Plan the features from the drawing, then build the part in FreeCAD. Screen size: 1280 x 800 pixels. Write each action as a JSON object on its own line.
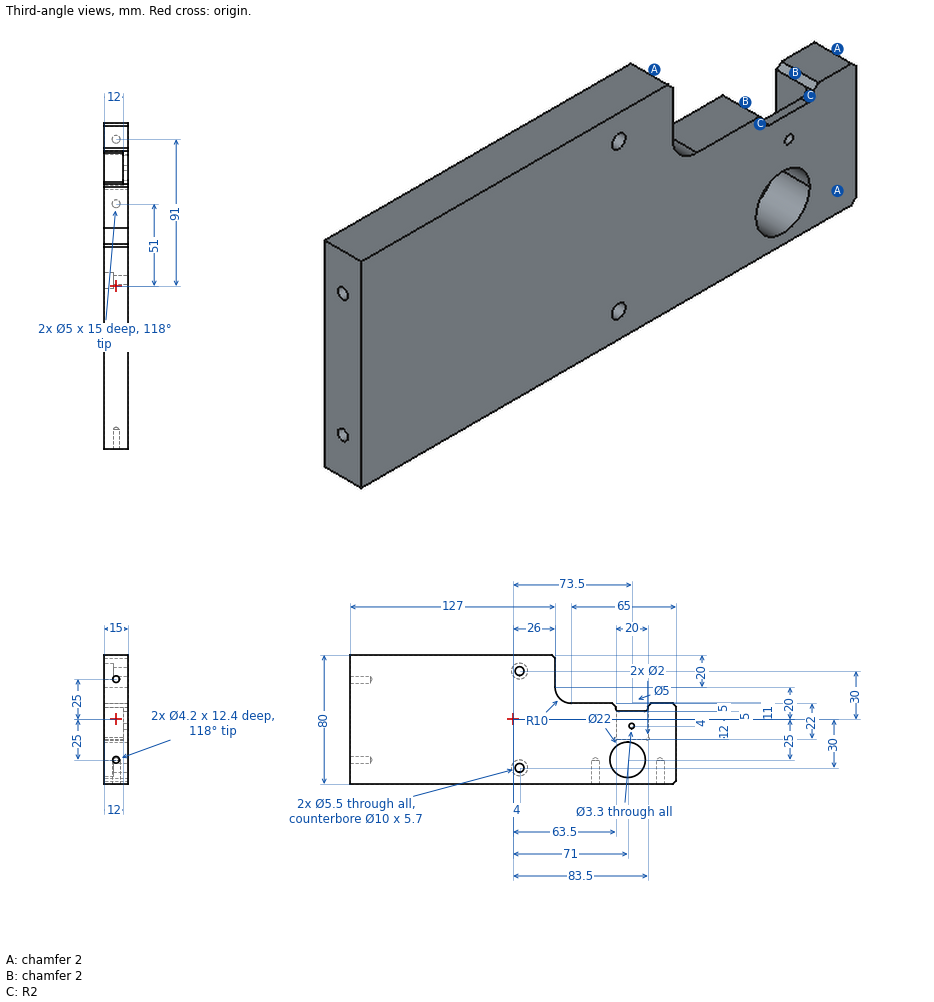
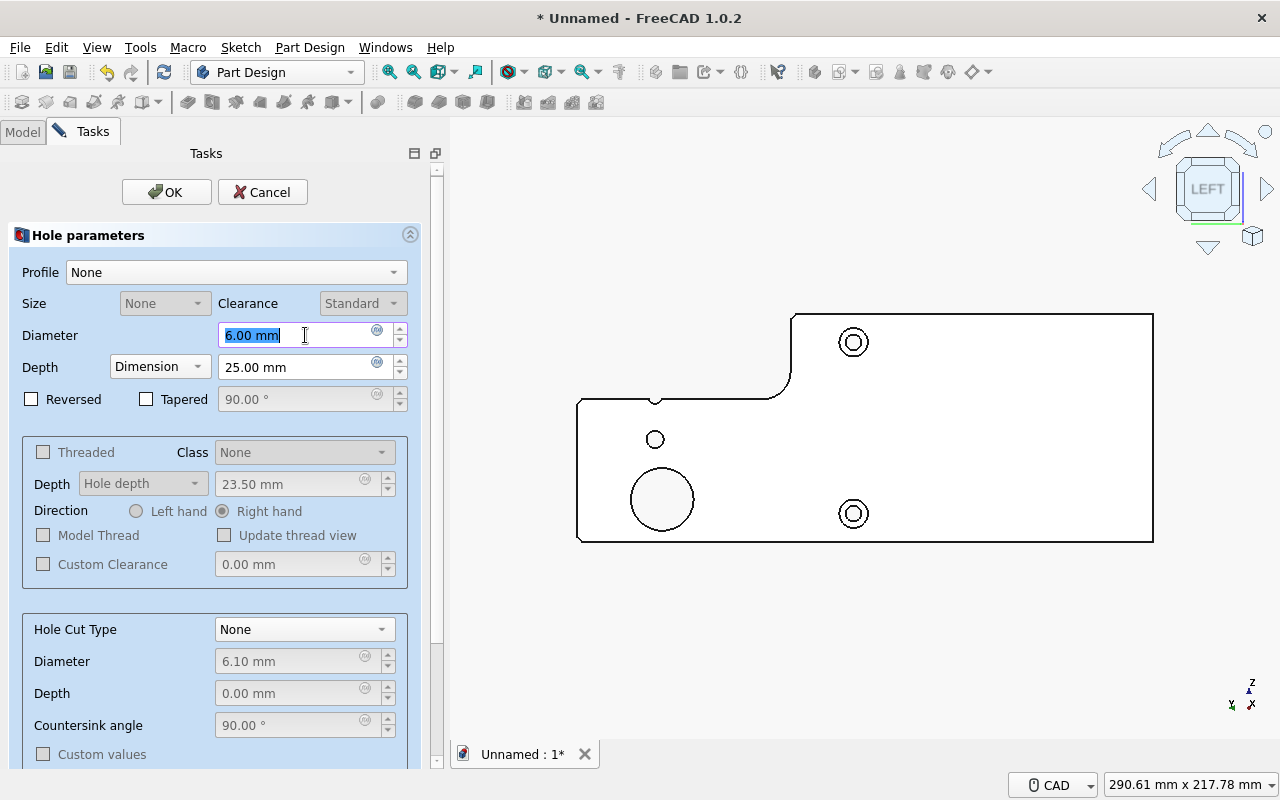
{"action": "type", "text": "3.3"}
{"action": "key", "text": "Tab"}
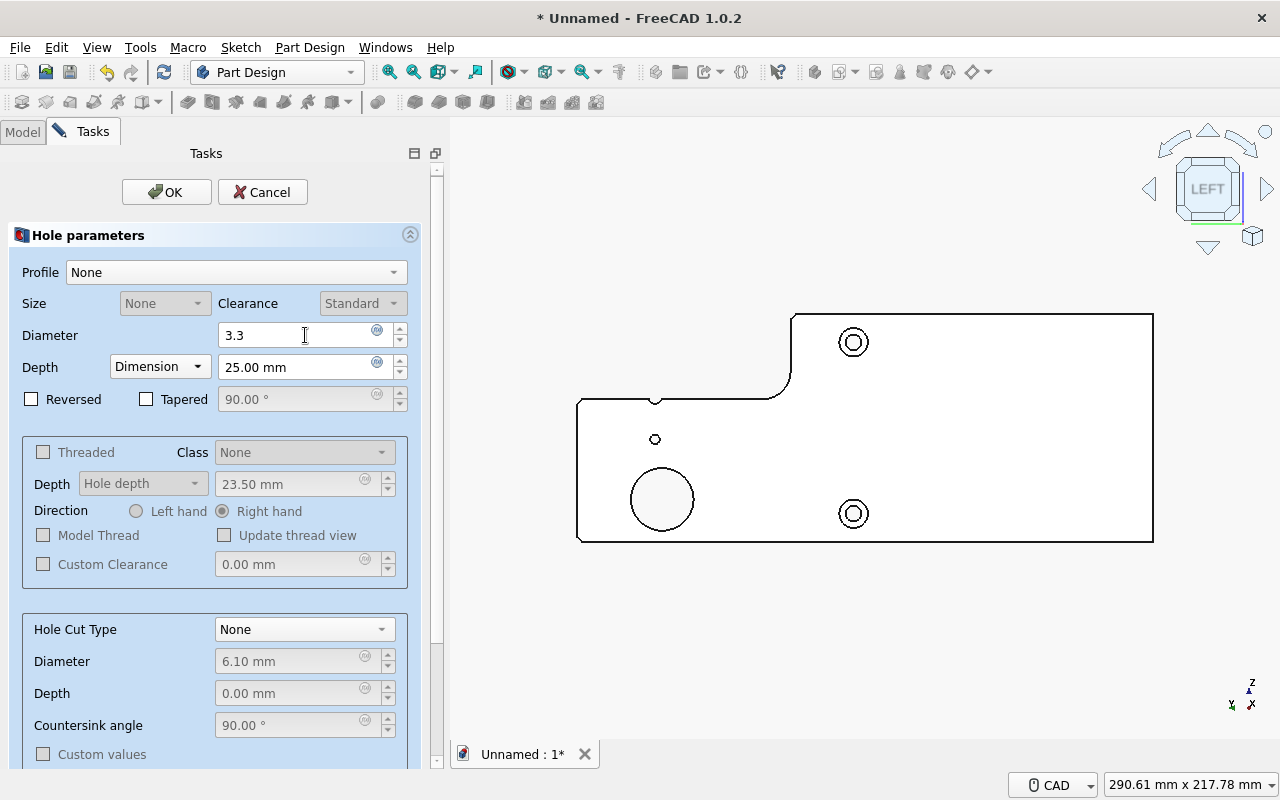
{"action": "left_click", "coordinate": [161, 366]}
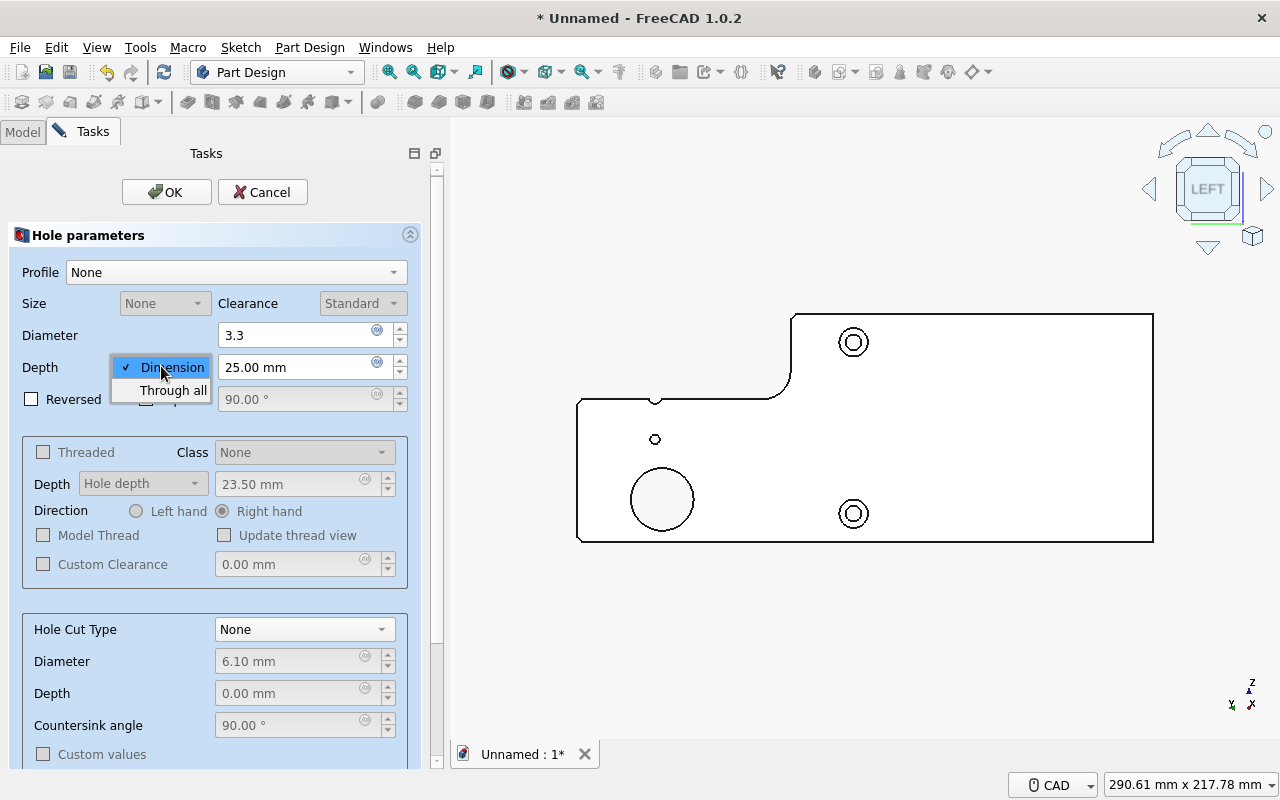
{"action": "left_click", "coordinate": [160, 390]}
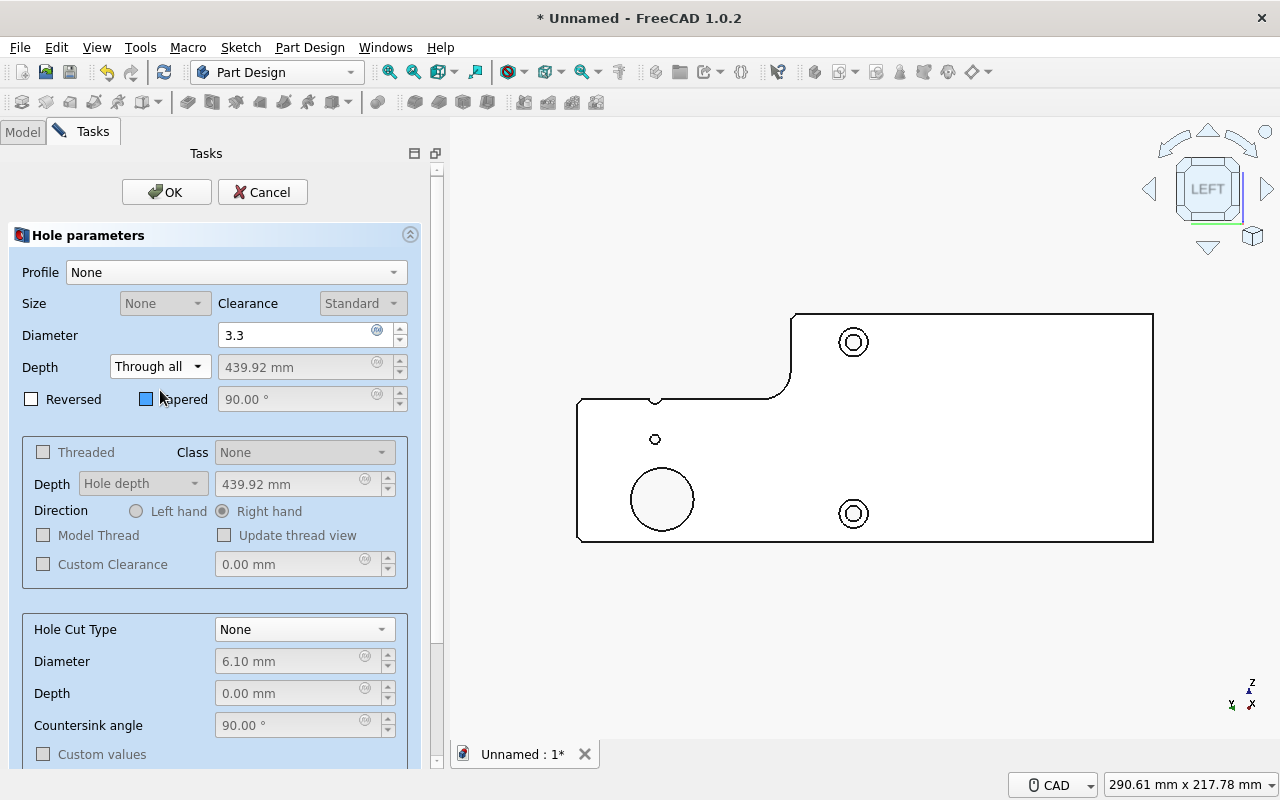
{"action": "left_click", "coordinate": [167, 192]}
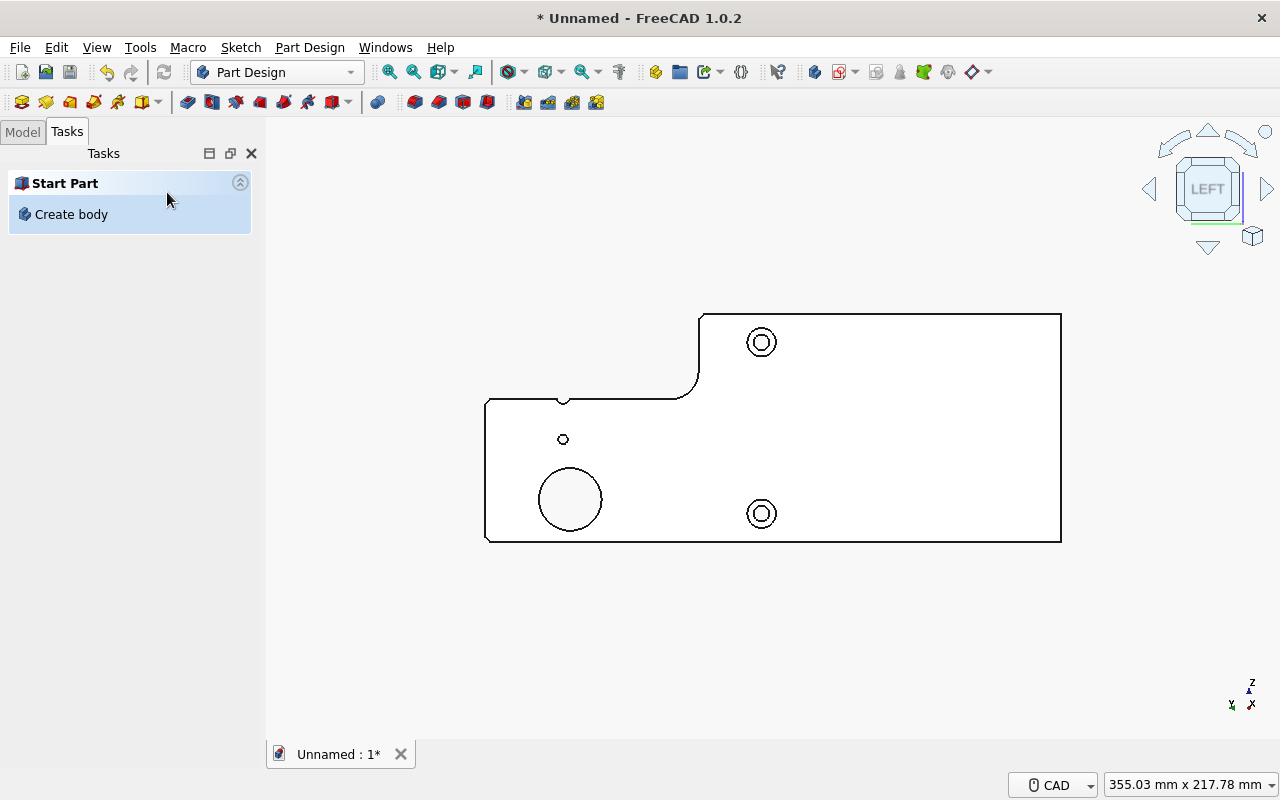
{"action": "left_click", "coordinate": [938, 427]}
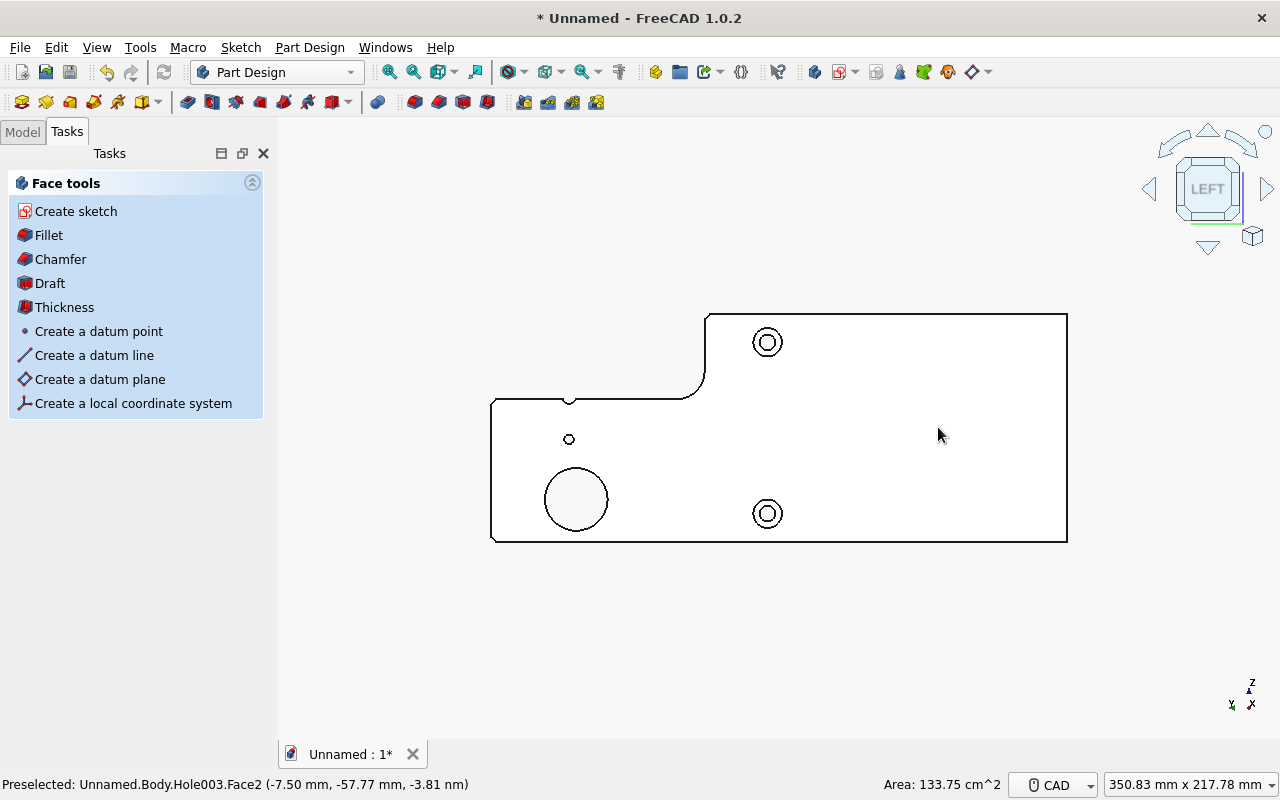
{"action": "left_click", "coordinate": [840, 72]}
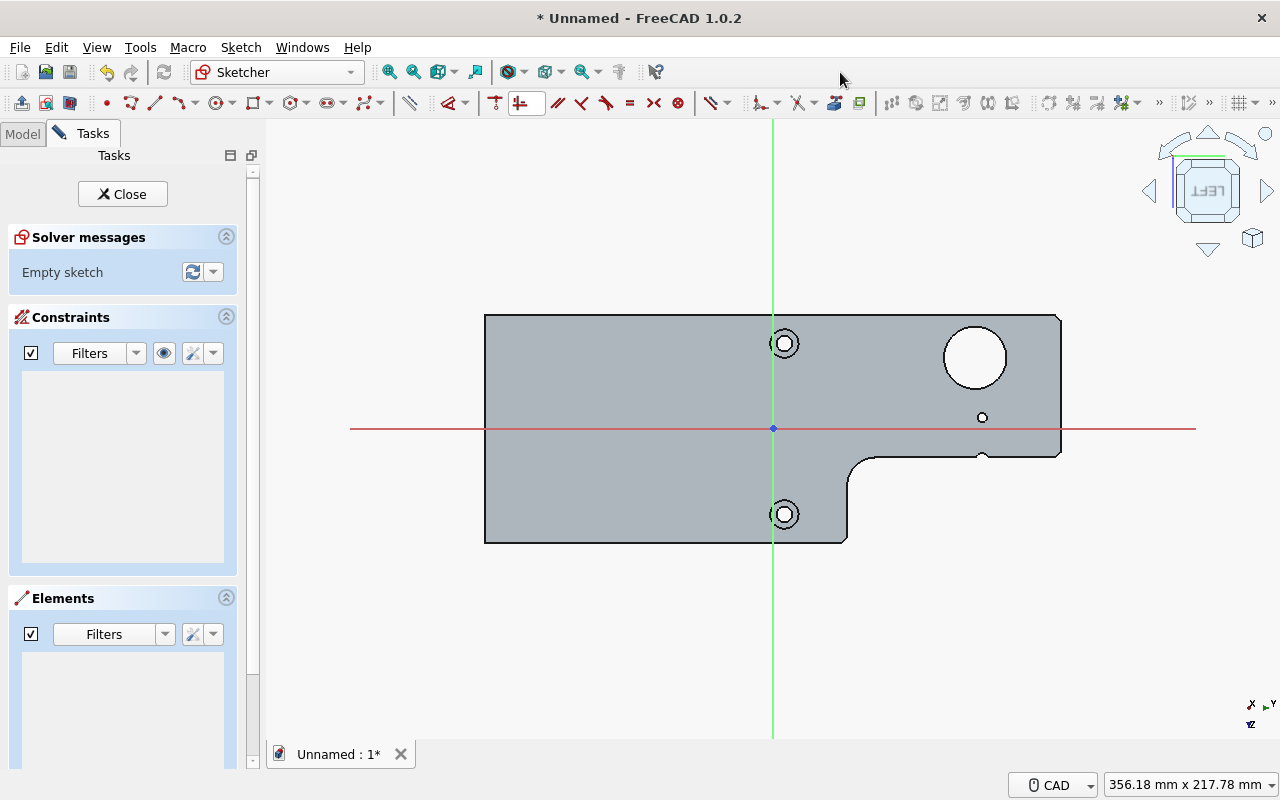
{"action": "scroll", "coordinate": [1037, 426], "scroll_direction": "up", "scroll_amount": 9}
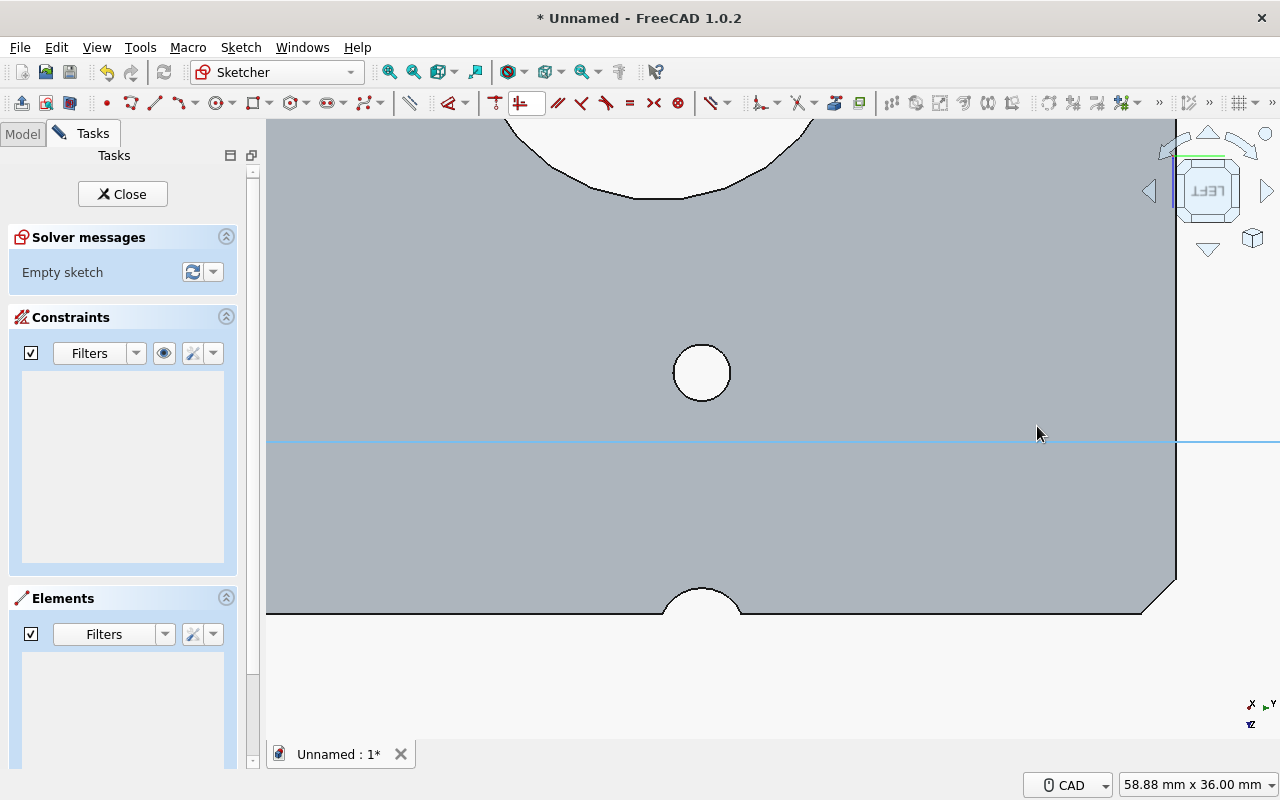
{"action": "left_click", "coordinate": [254, 104]}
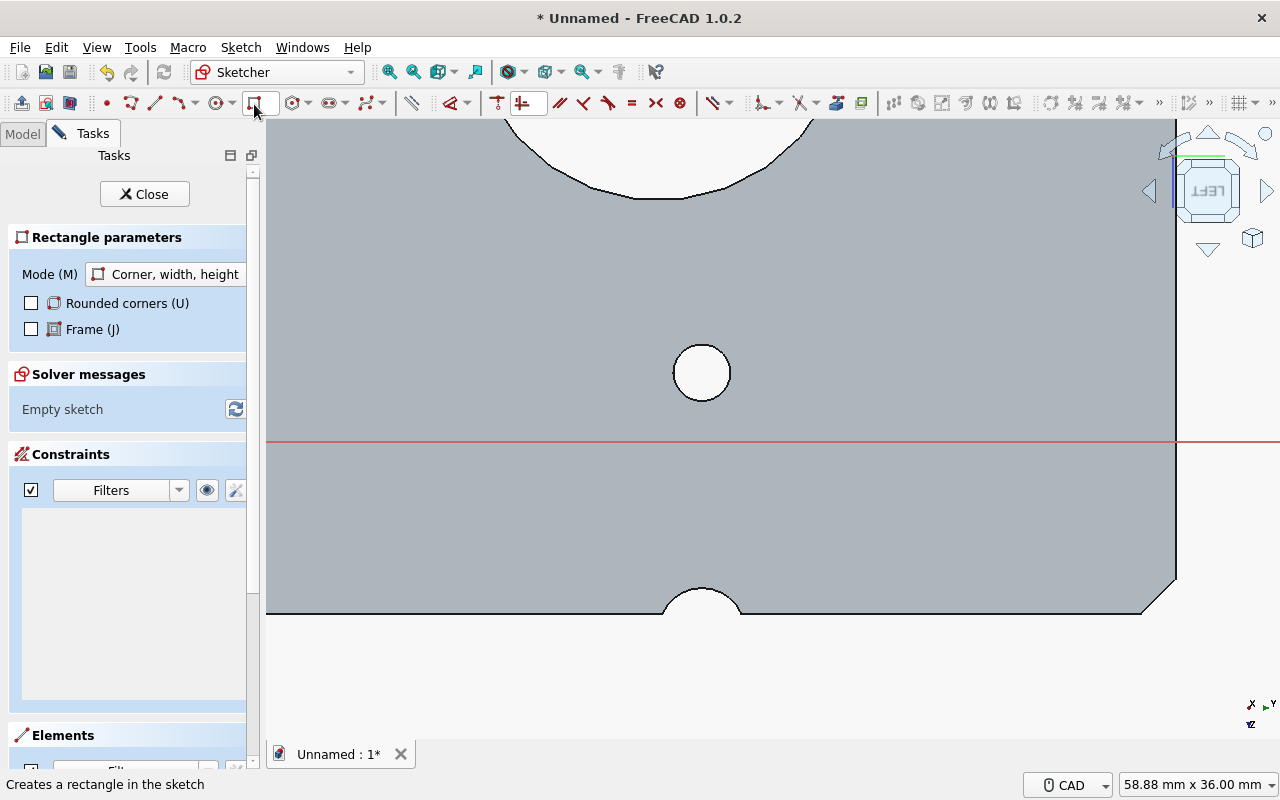
{"action": "left_click", "coordinate": [530, 235]}
{"action": "left_click", "coordinate": [874, 614]}
{"action": "key", "text": "Escape"}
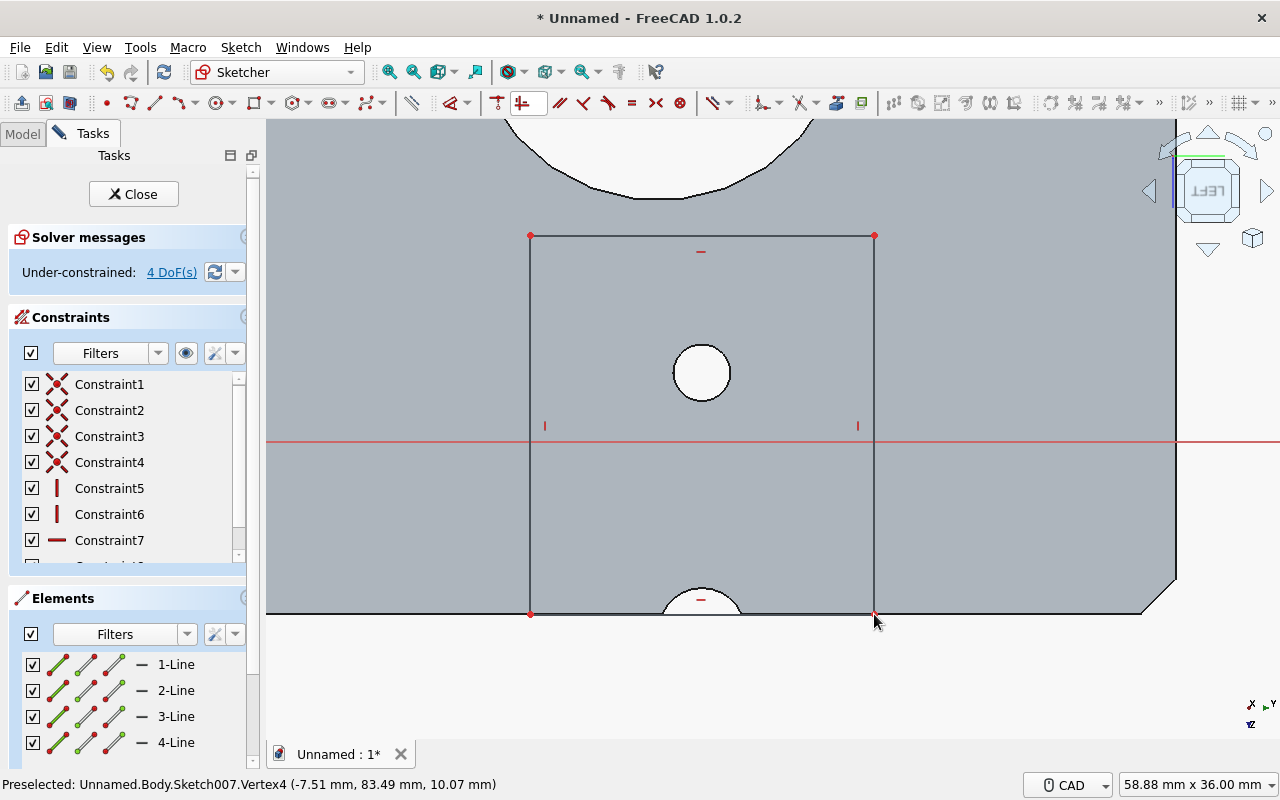
{"action": "left_click", "coordinate": [450, 104]}